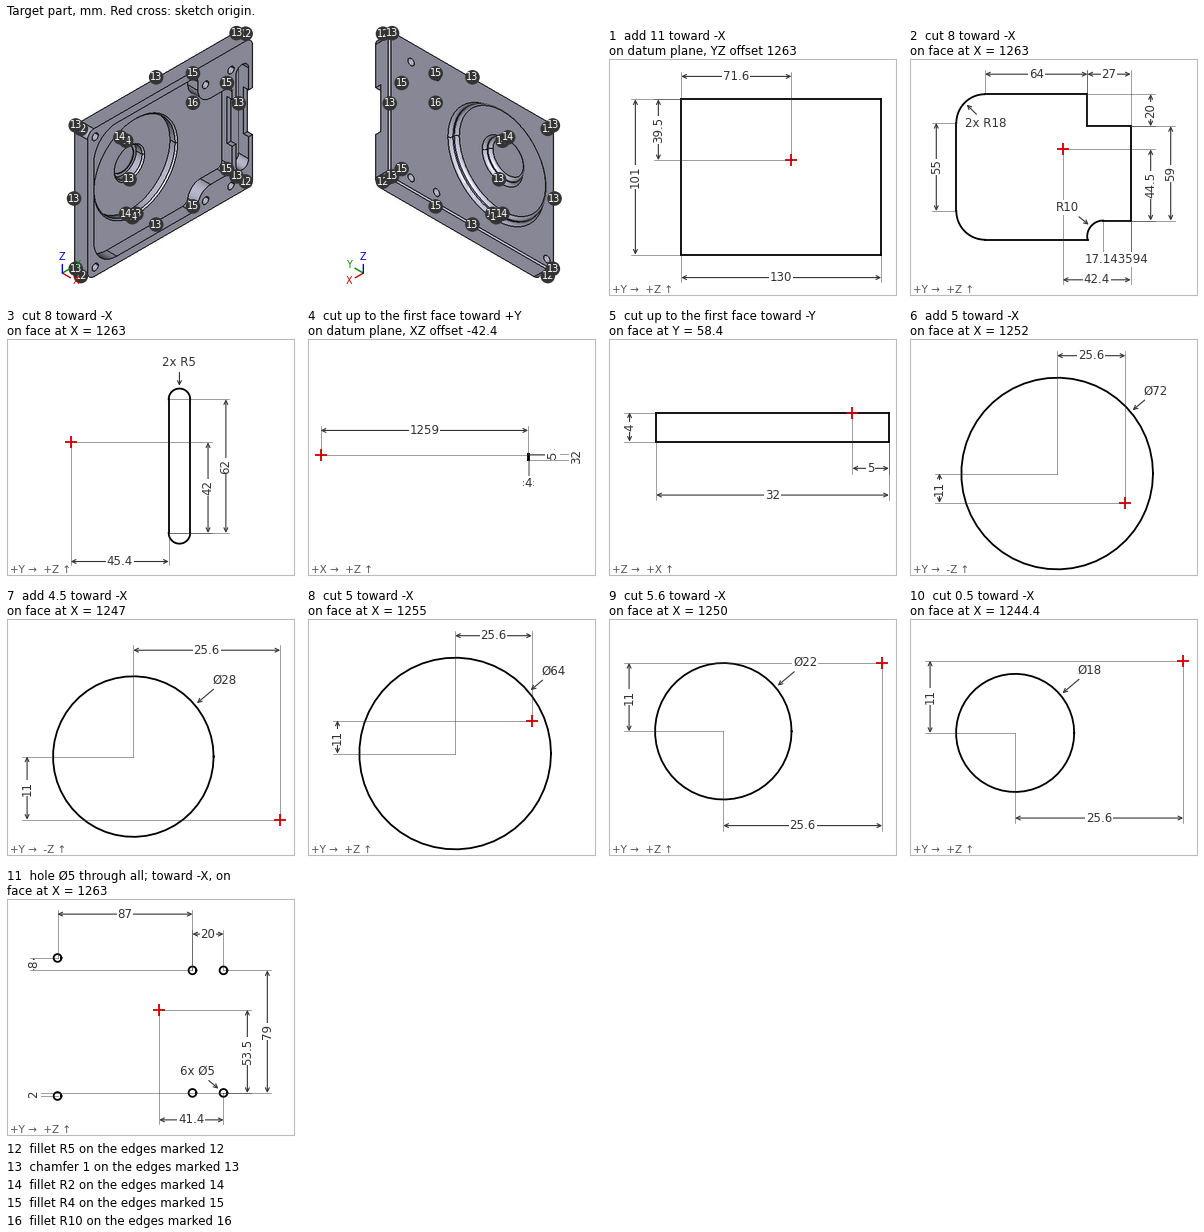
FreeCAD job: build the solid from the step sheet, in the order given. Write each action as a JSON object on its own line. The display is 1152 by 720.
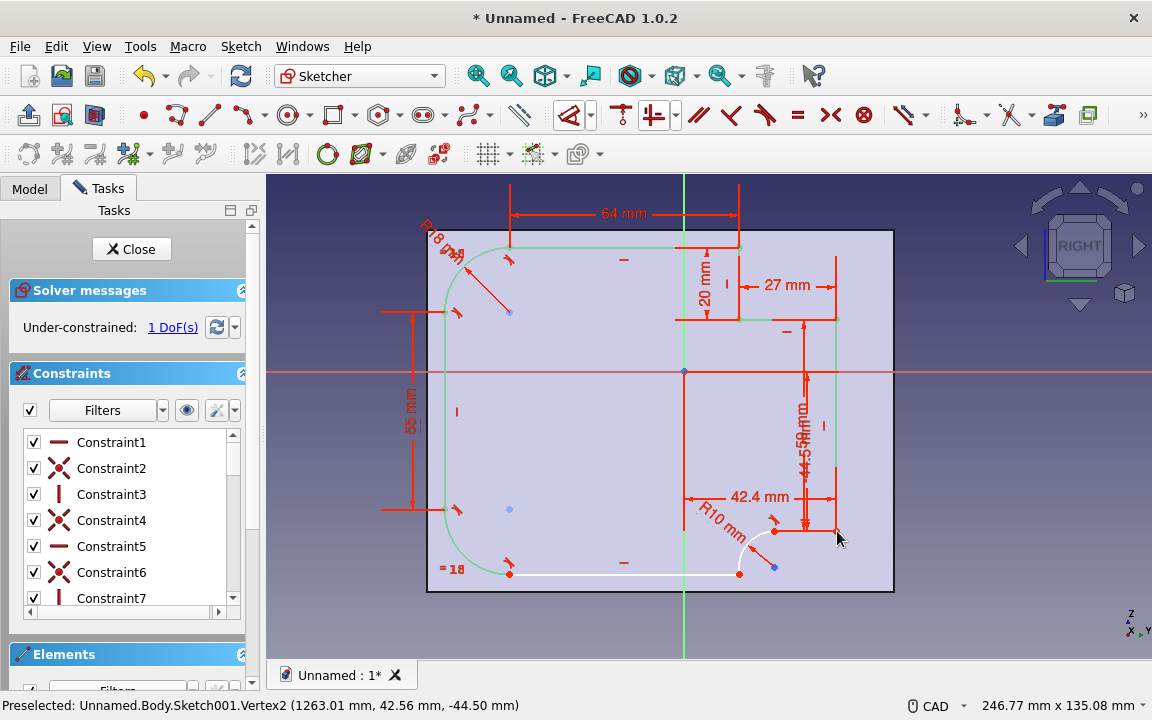
{"action": "left_click", "coordinate": [793, 531]}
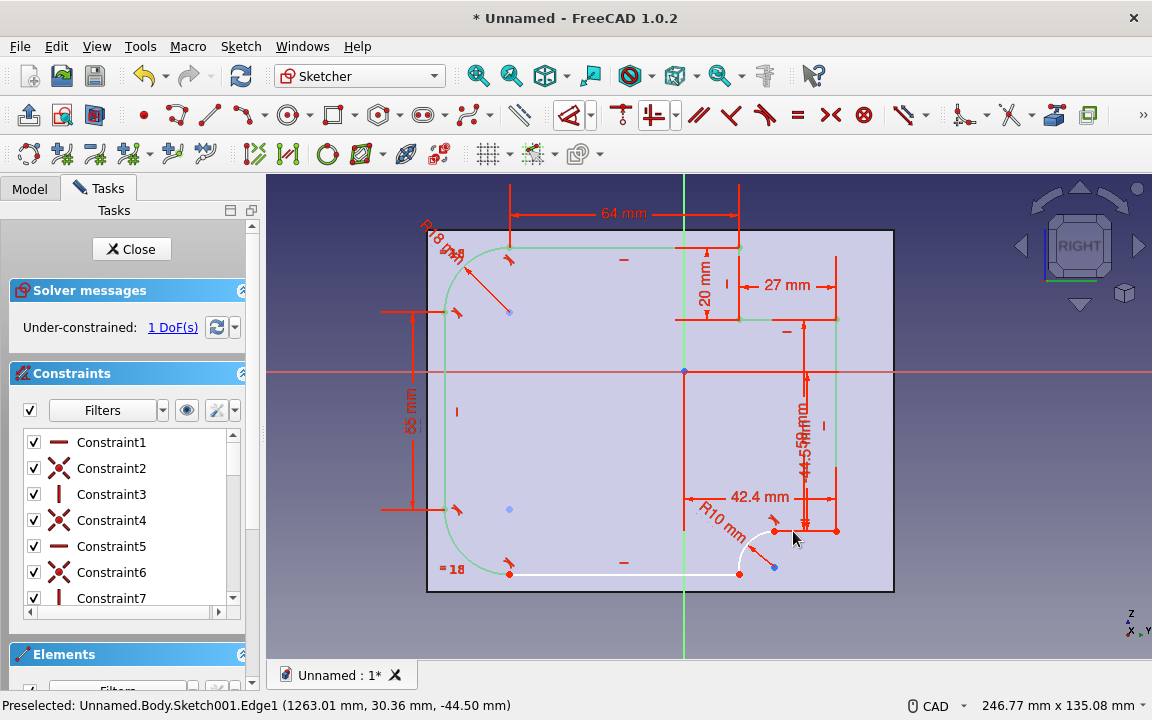
{"action": "left_click", "coordinate": [590, 116]}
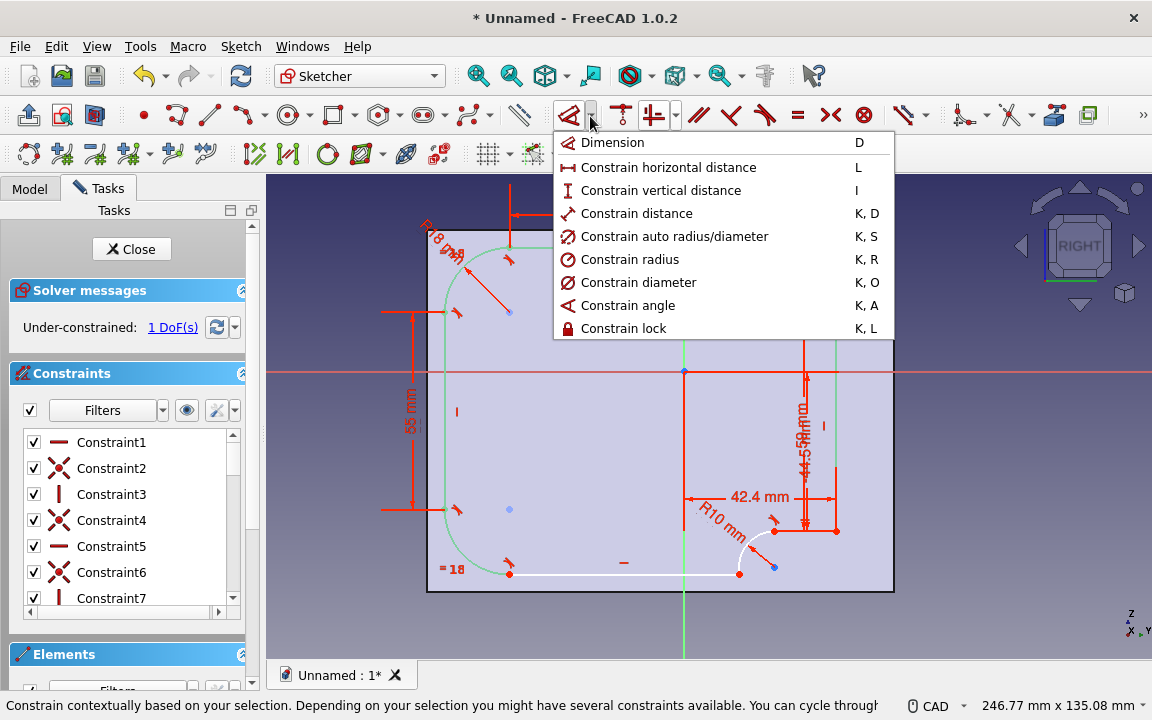
{"action": "left_click", "coordinate": [724, 168]}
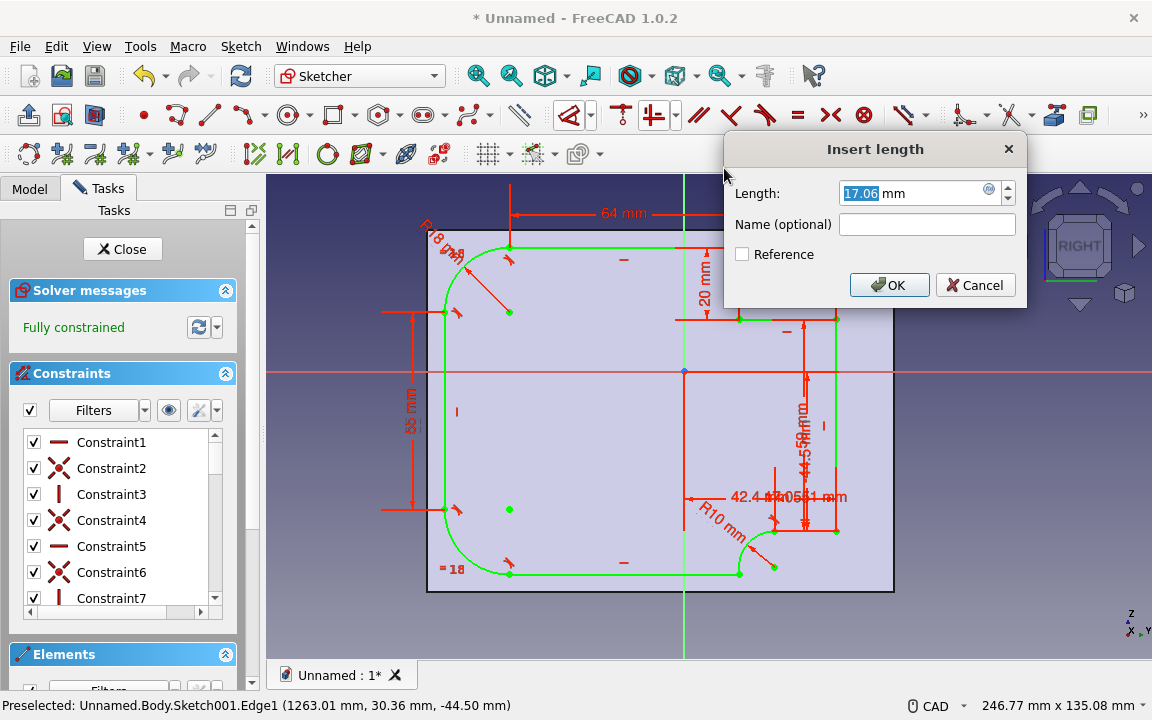
{"action": "type", "text": "17.143594"}
{"action": "key", "text": "Return"}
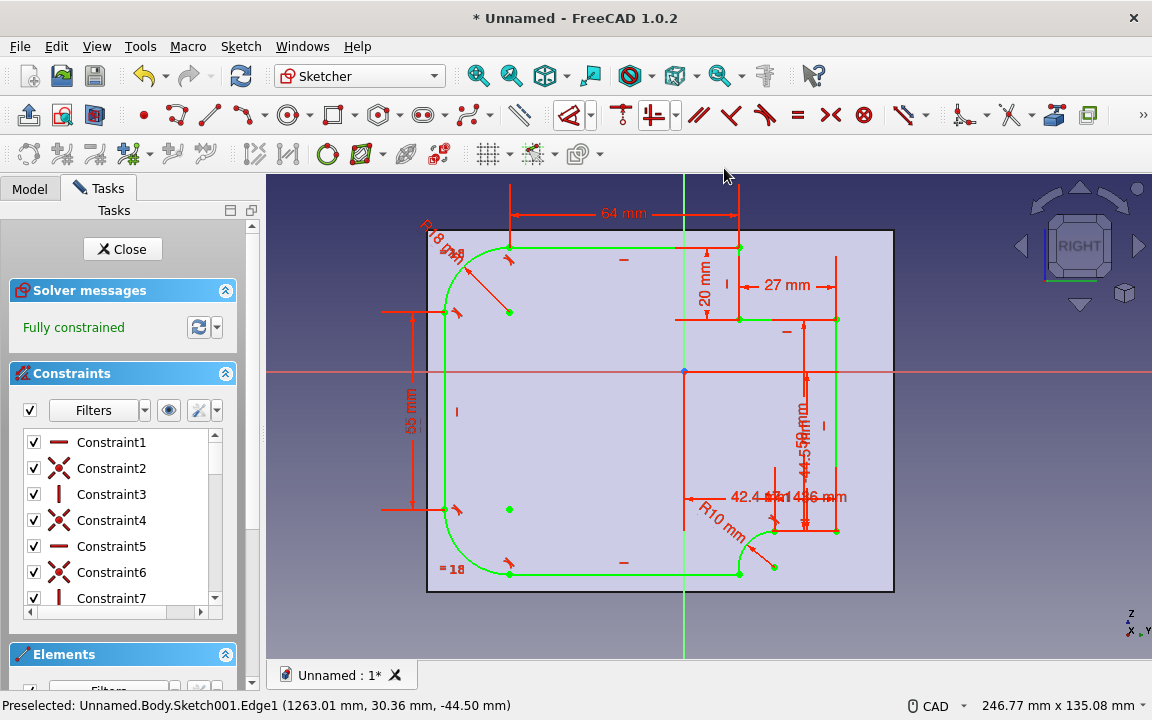
{"action": "left_click", "coordinate": [123, 249]}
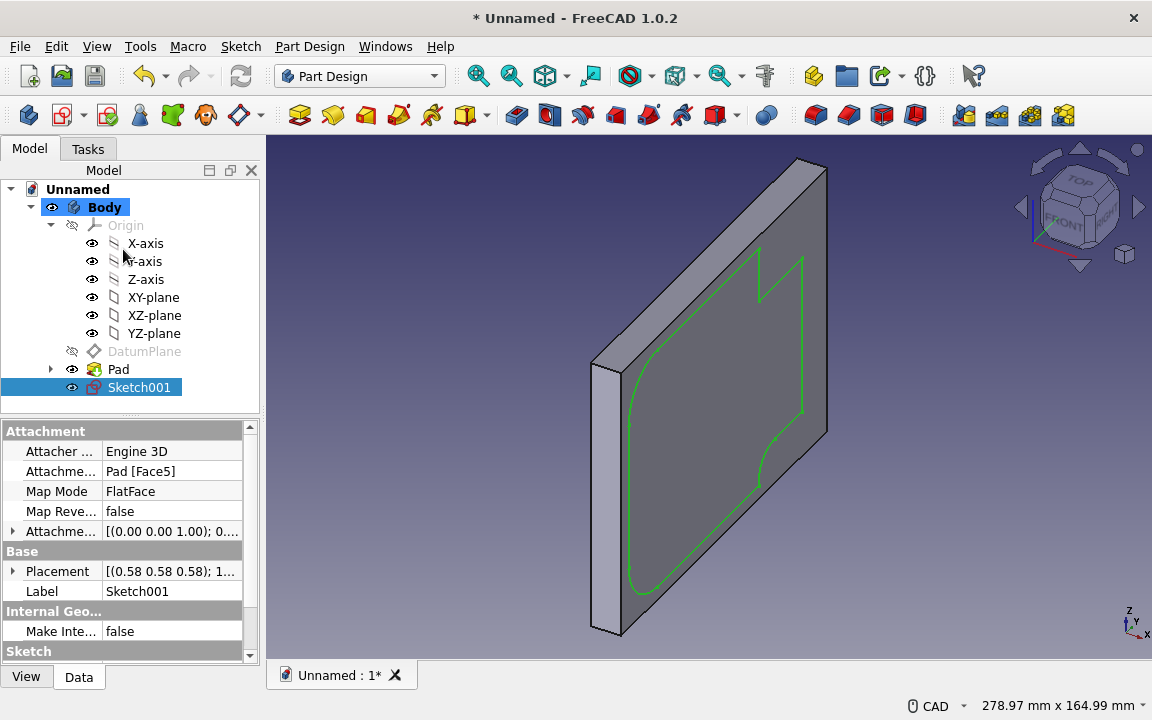
{"action": "left_click", "coordinate": [517, 116]}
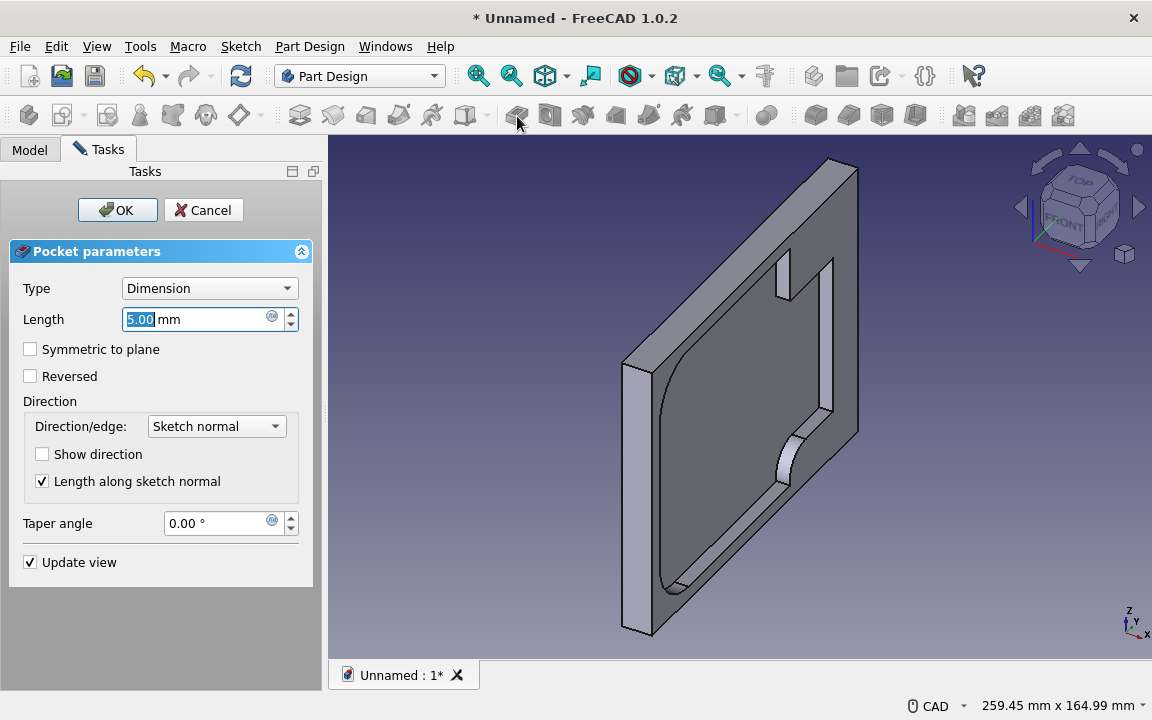
{"action": "type", "text": "8"}
{"action": "key", "text": "Tab"}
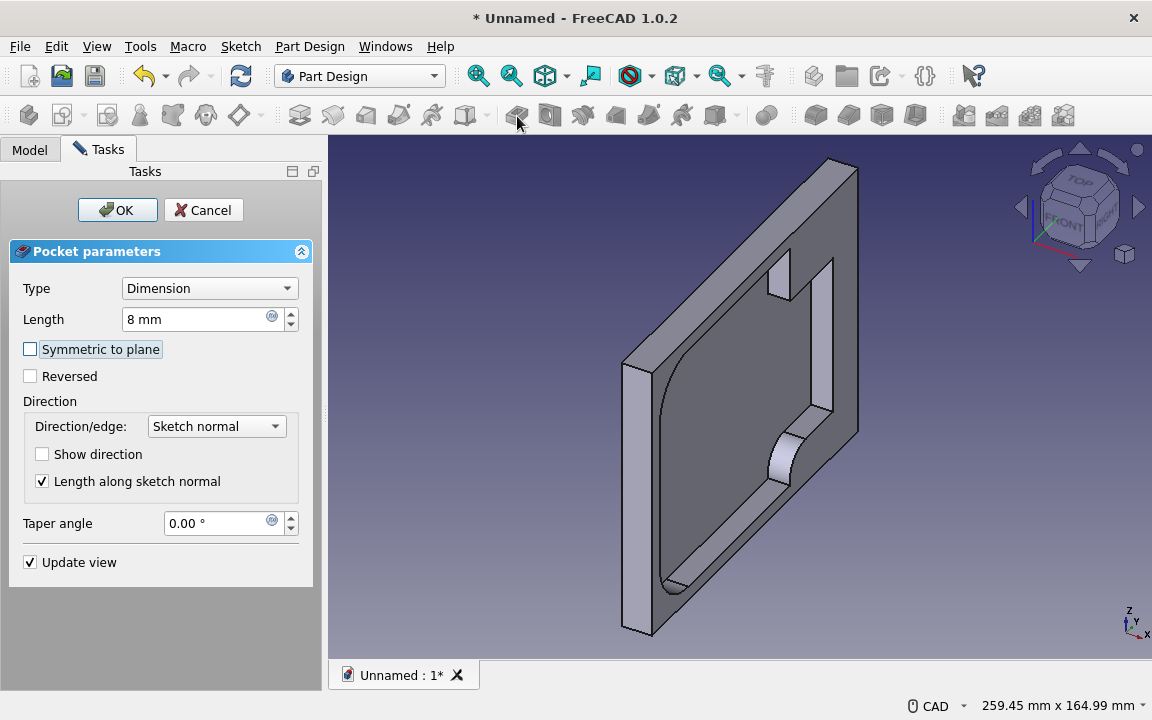
{"action": "left_click", "coordinate": [118, 210]}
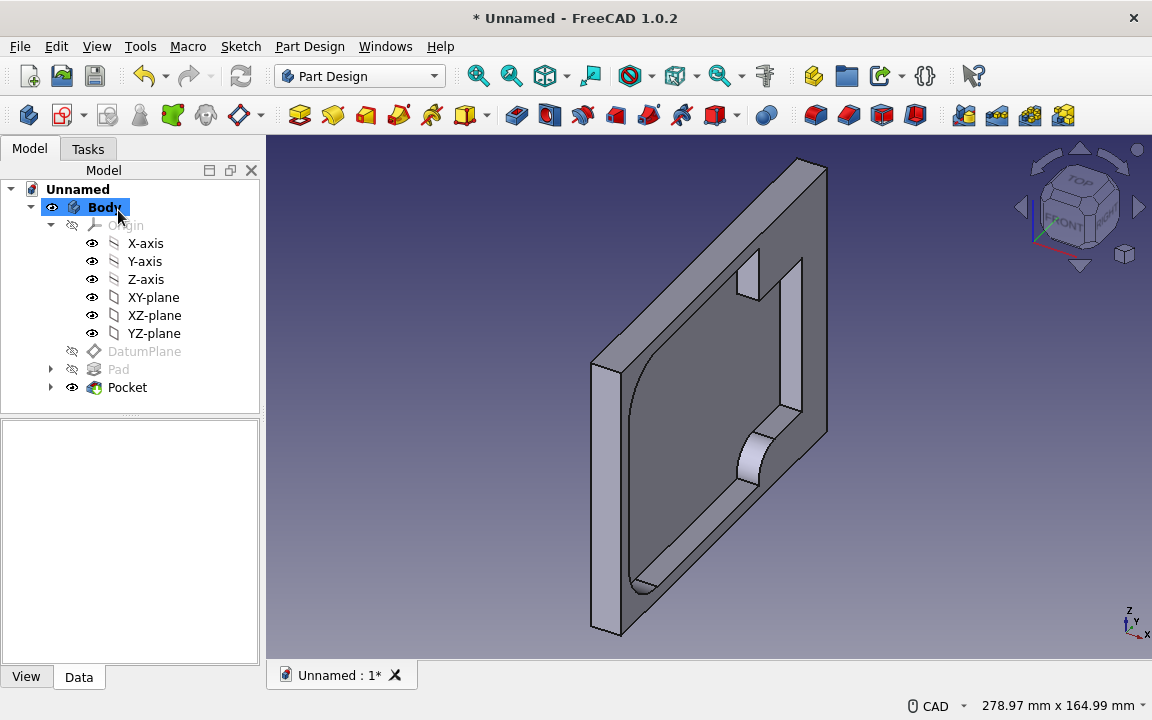
{"action": "left_click", "coordinate": [813, 238]}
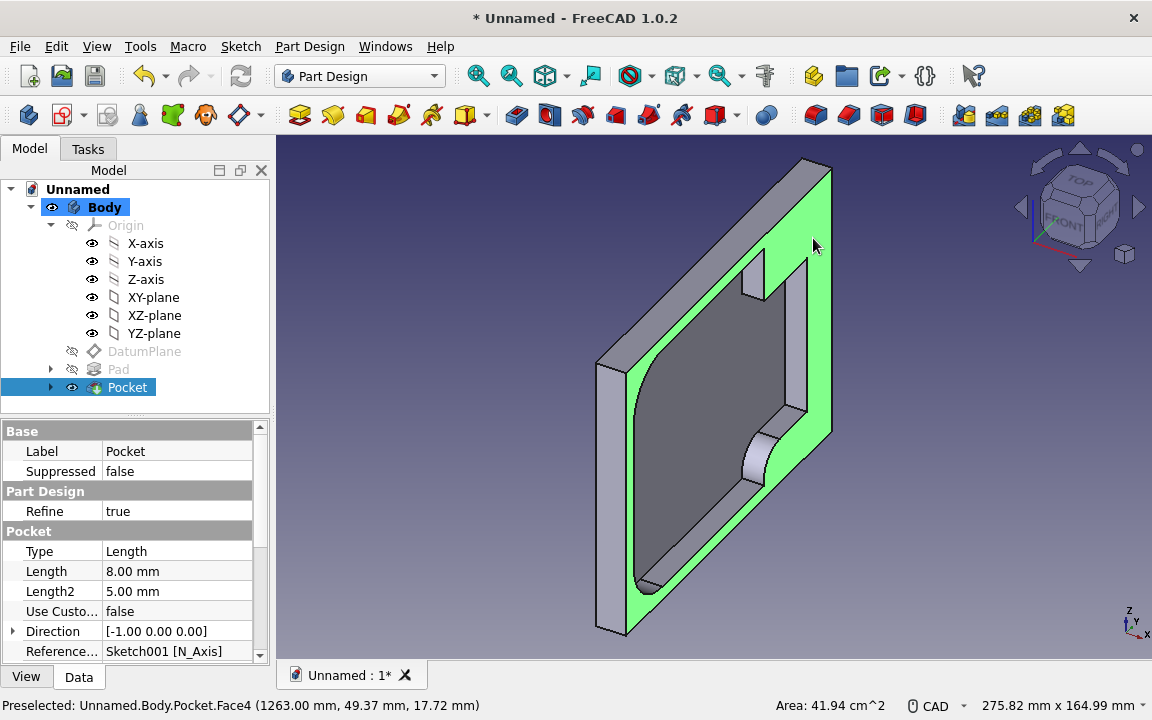
{"action": "left_click", "coordinate": [62, 116]}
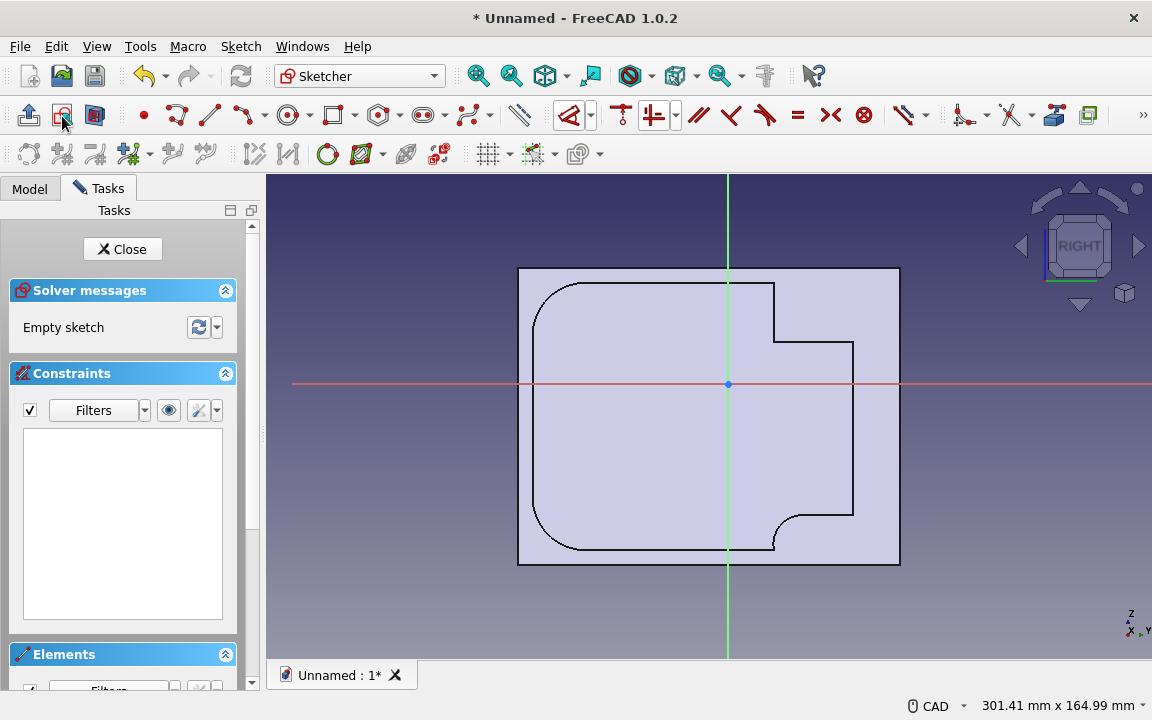
{"action": "scroll", "coordinate": [987, 417], "scroll_direction": "up", "scroll_amount": 2}